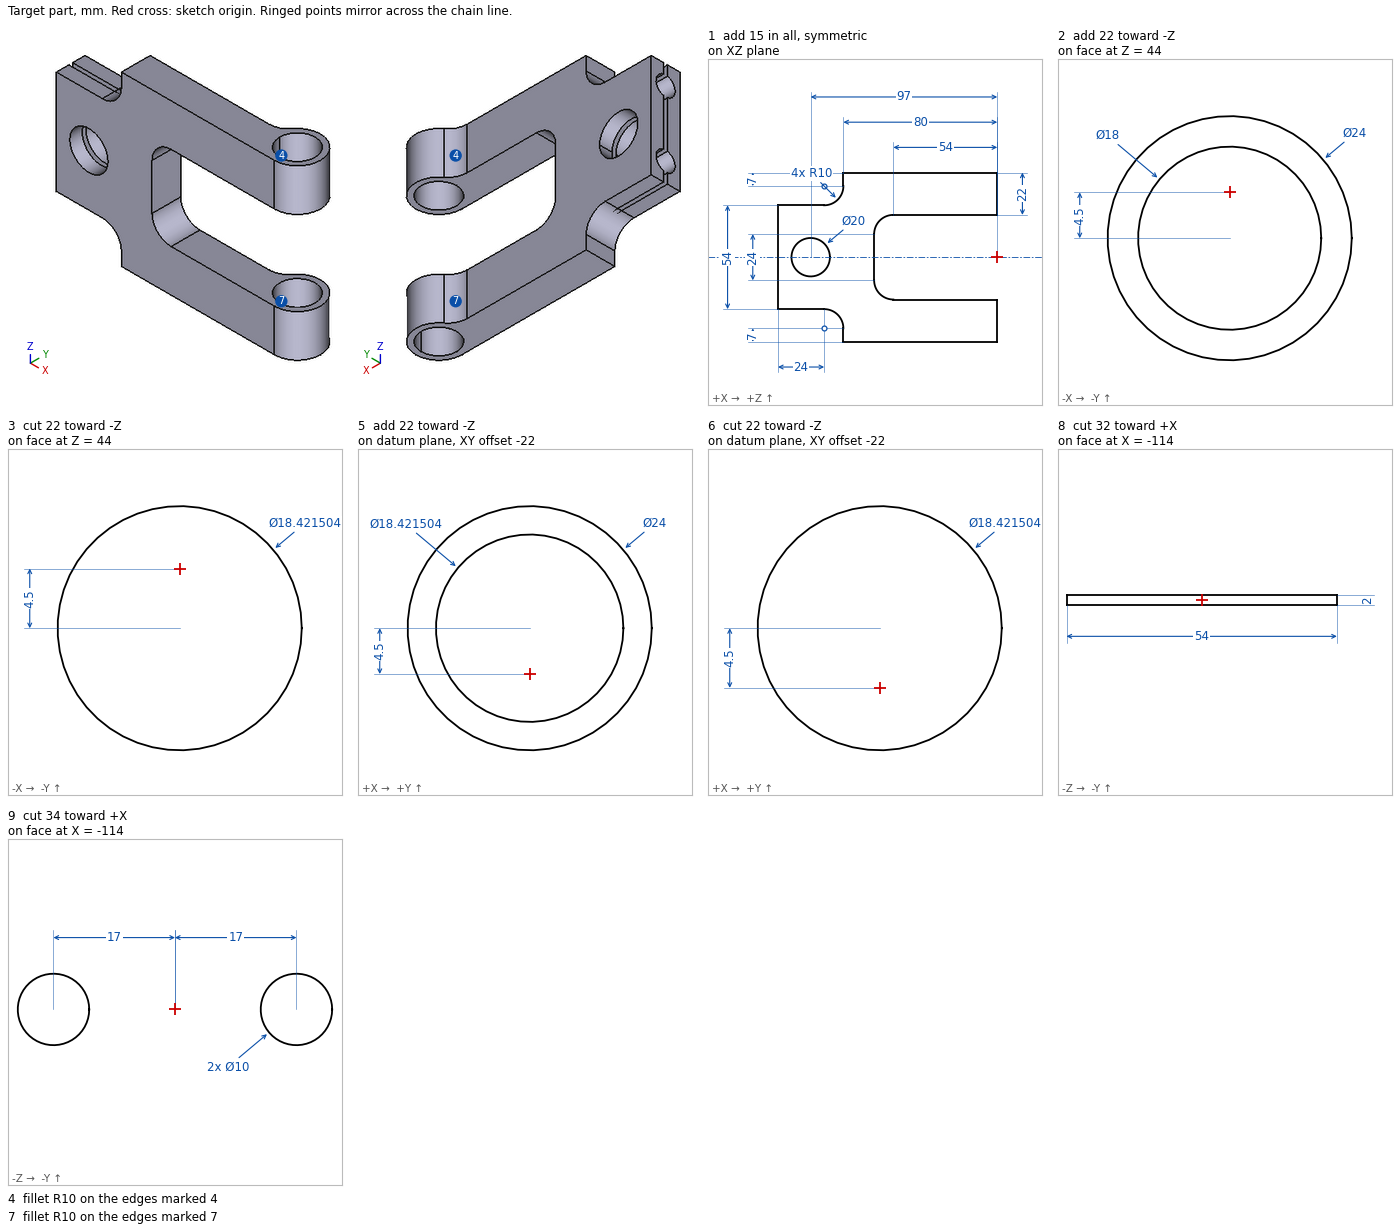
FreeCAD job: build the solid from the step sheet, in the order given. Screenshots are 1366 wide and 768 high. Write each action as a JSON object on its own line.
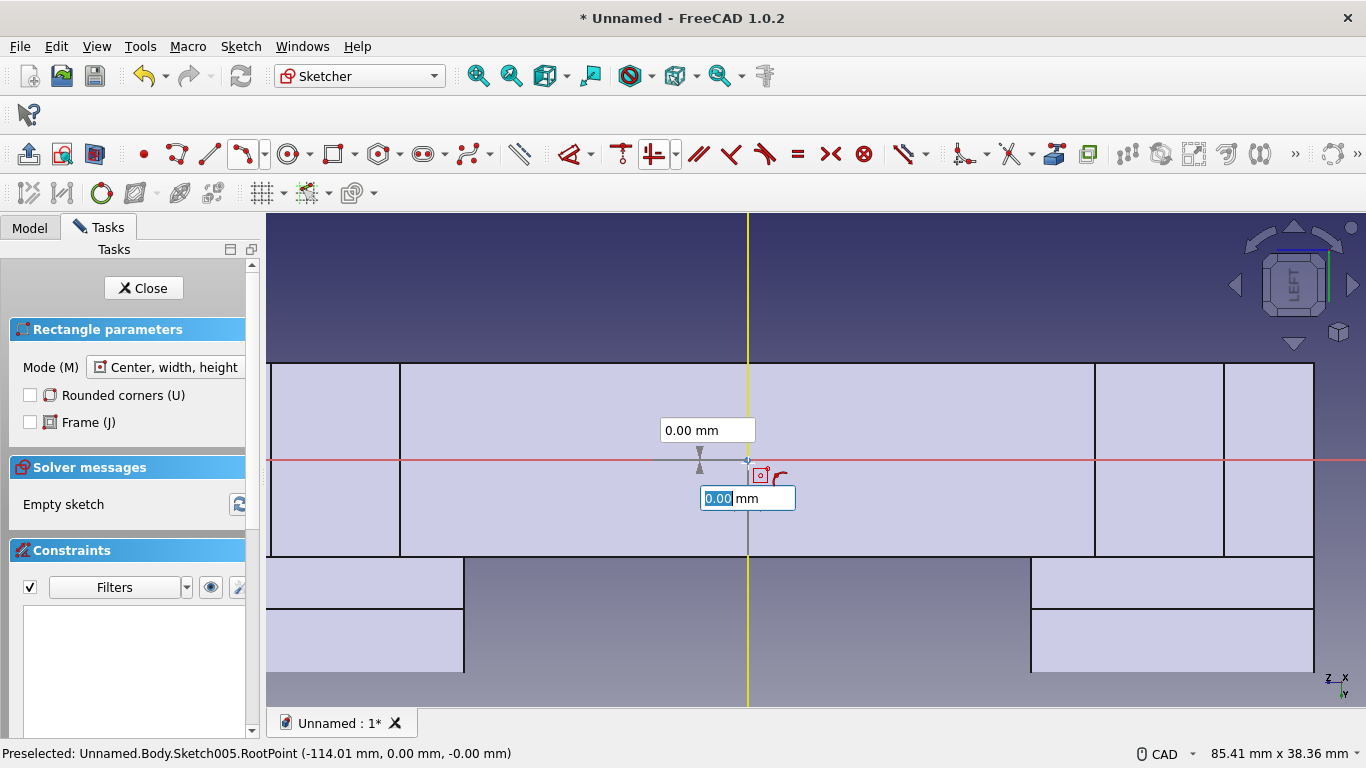
{"action": "scroll", "coordinate": [1095, 447], "scroll_direction": "up", "scroll_amount": 2}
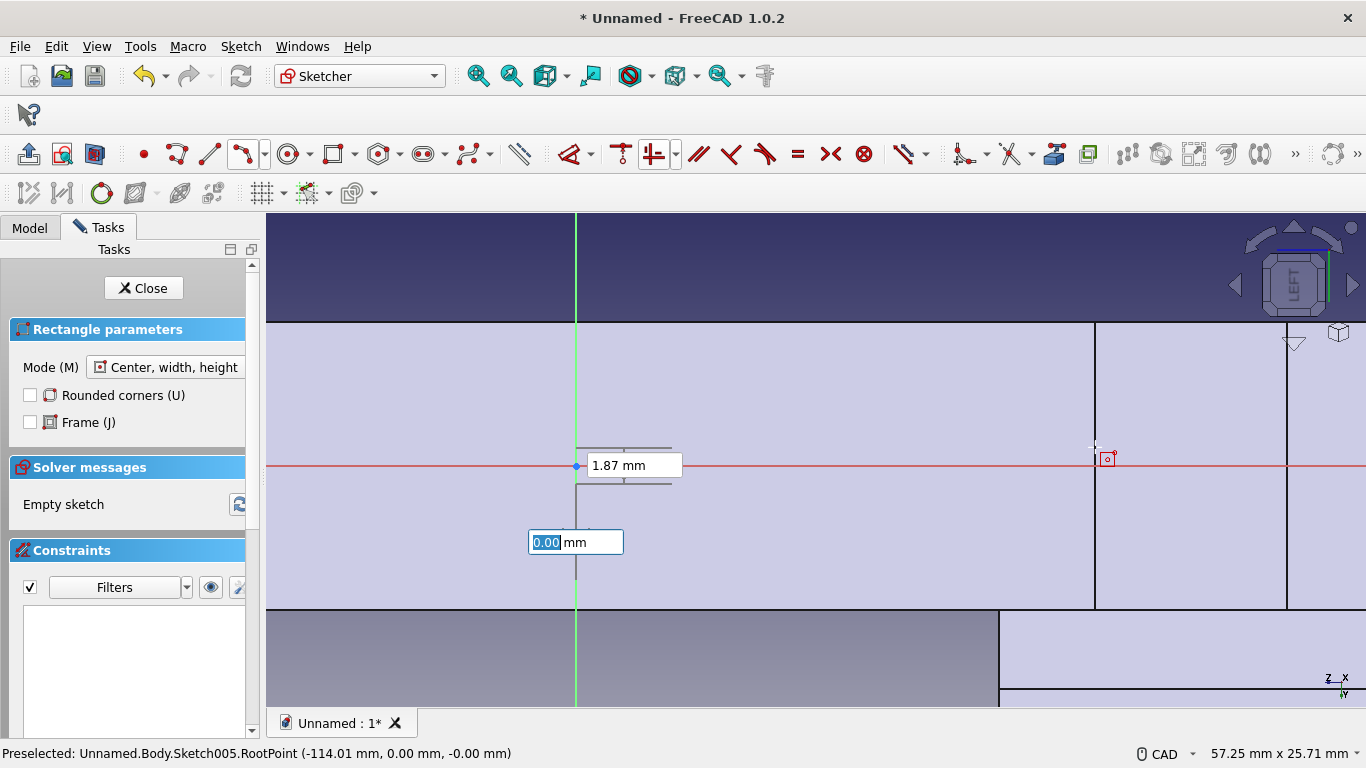
{"action": "left_click", "coordinate": [1095, 447]}
{"action": "key", "text": "Escape"}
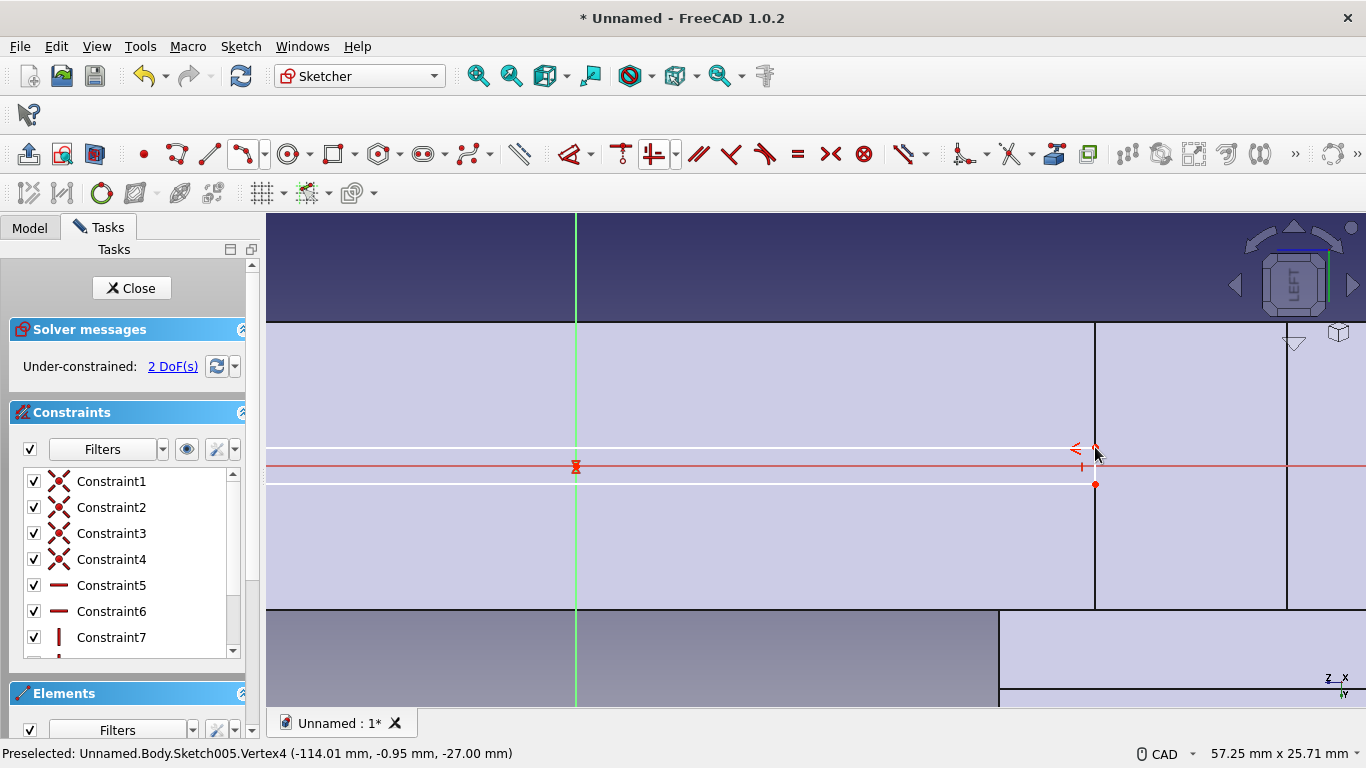
{"action": "left_click", "coordinate": [568, 154]}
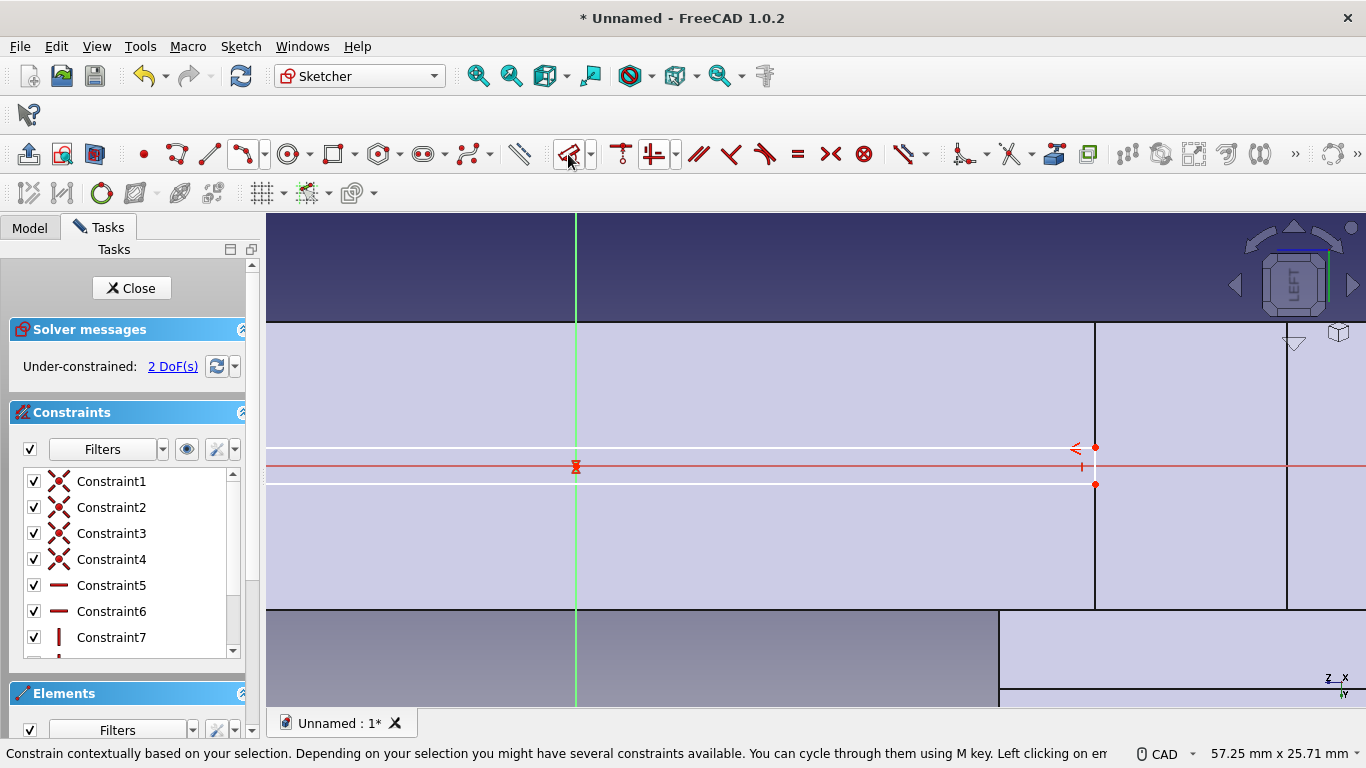
{"action": "left_click", "coordinate": [1095, 470]}
{"action": "left_click", "coordinate": [1129, 458]}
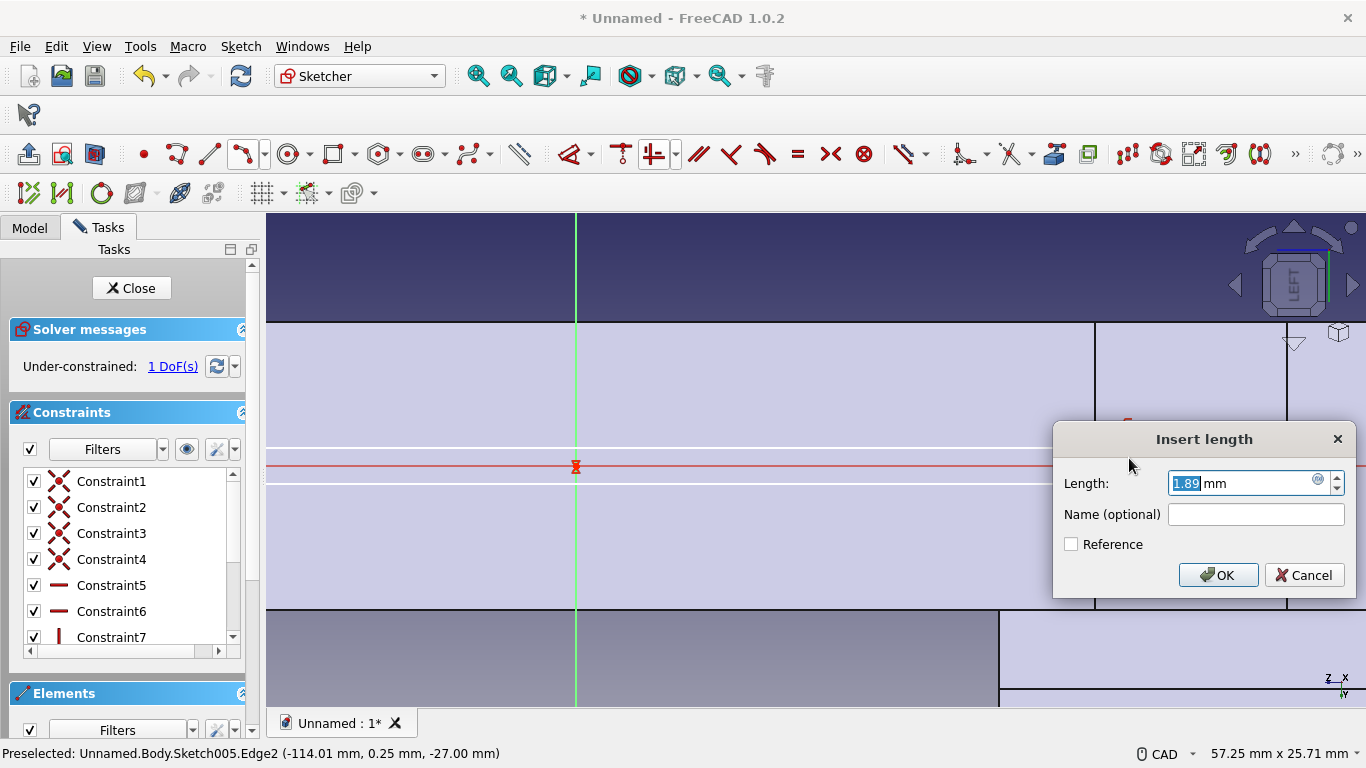
{"action": "type", "text": "2"}
{"action": "key", "text": "Return"}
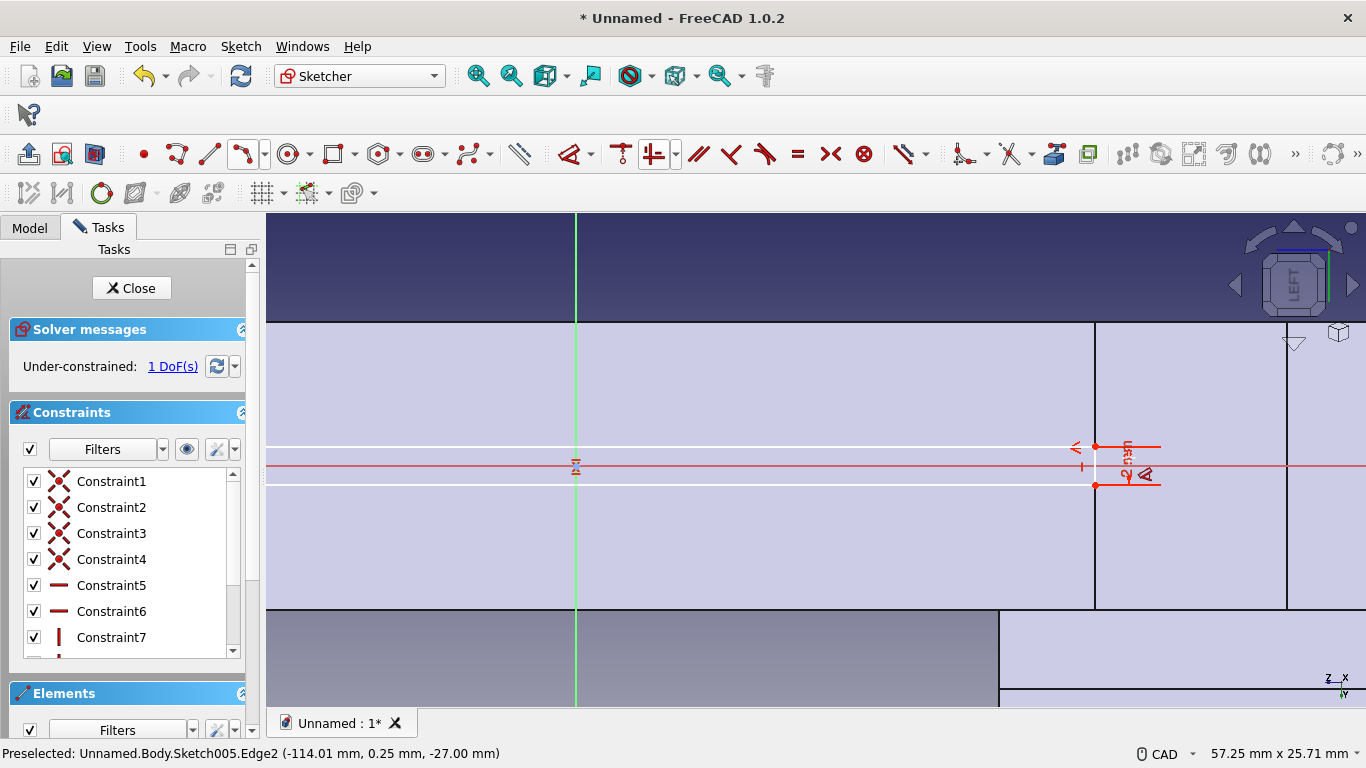
{"action": "left_click", "coordinate": [369, 485]}
{"action": "left_click", "coordinate": [695, 519]}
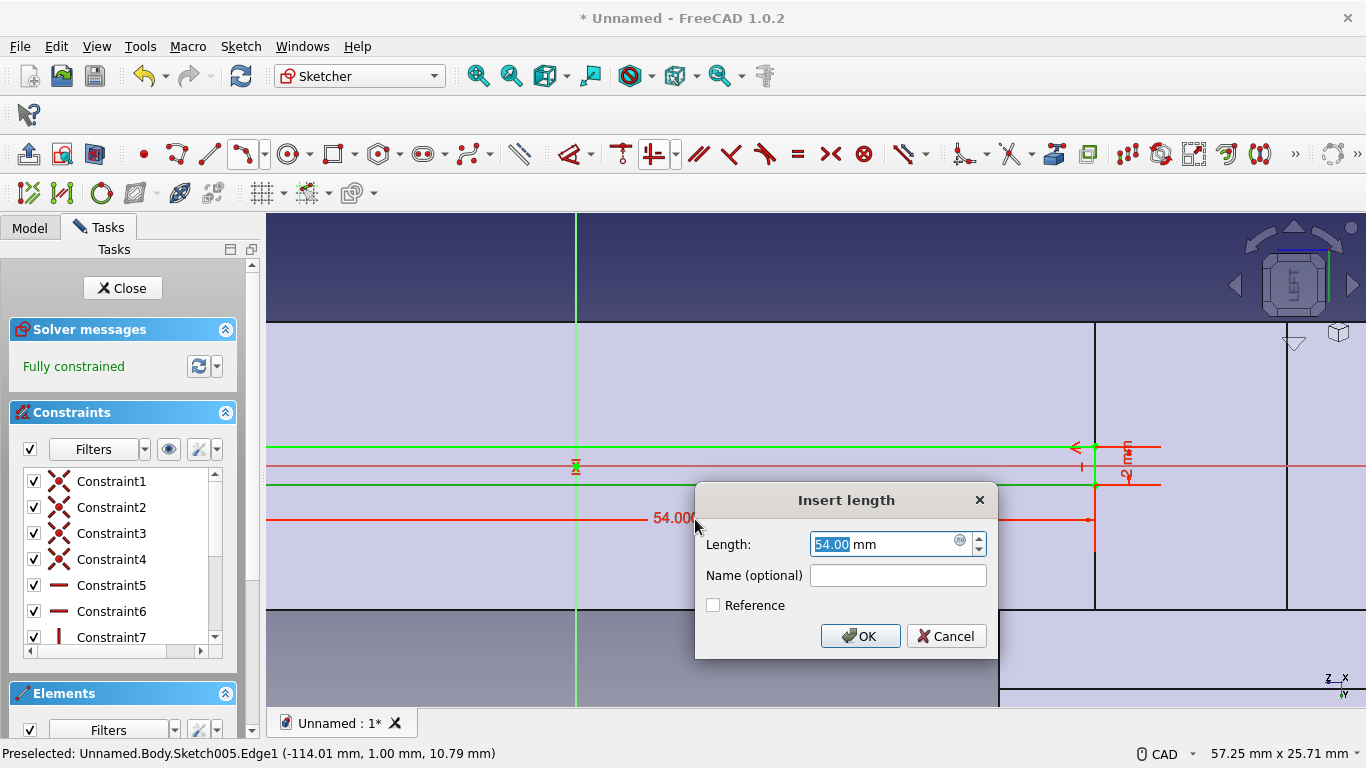
{"action": "type", "text": "54"}
{"action": "key", "text": "Return"}
{"action": "key", "text": "Escape"}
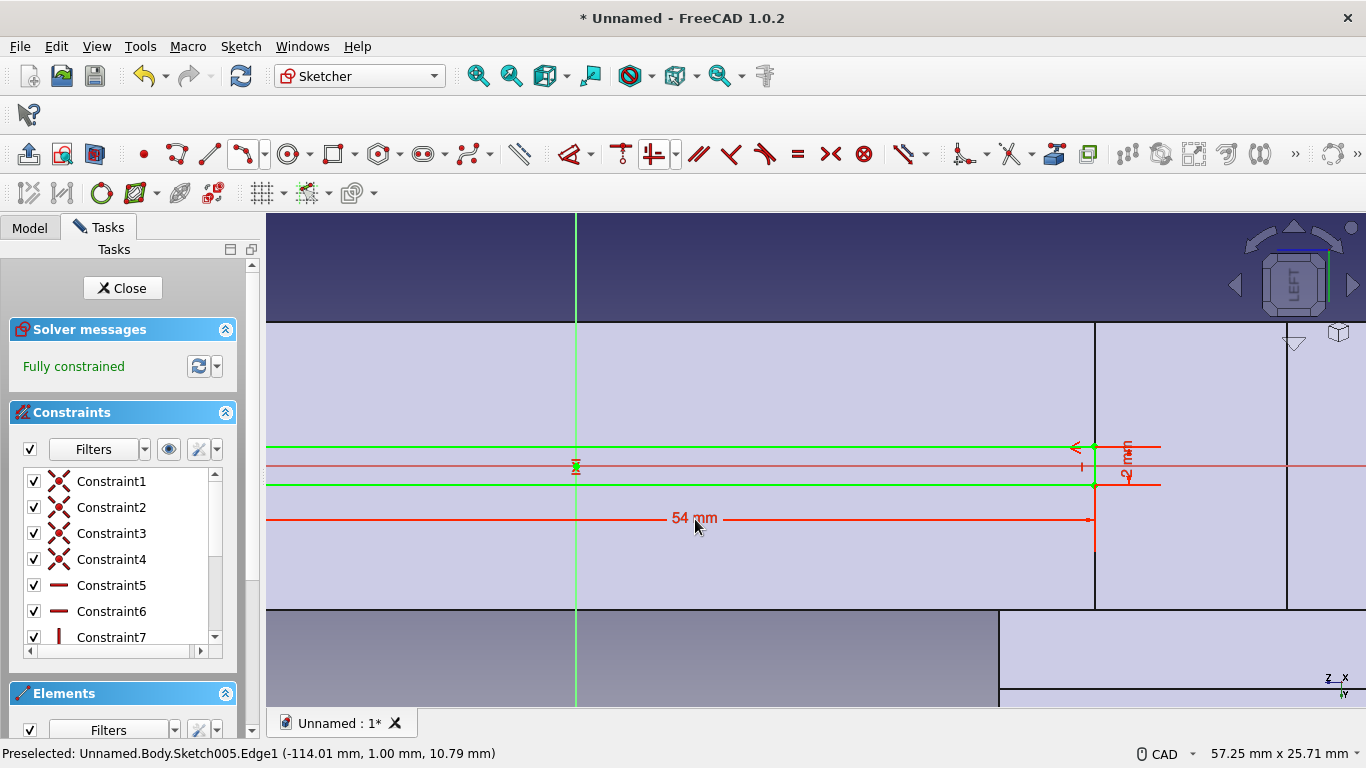
{"action": "left_click", "coordinate": [123, 288]}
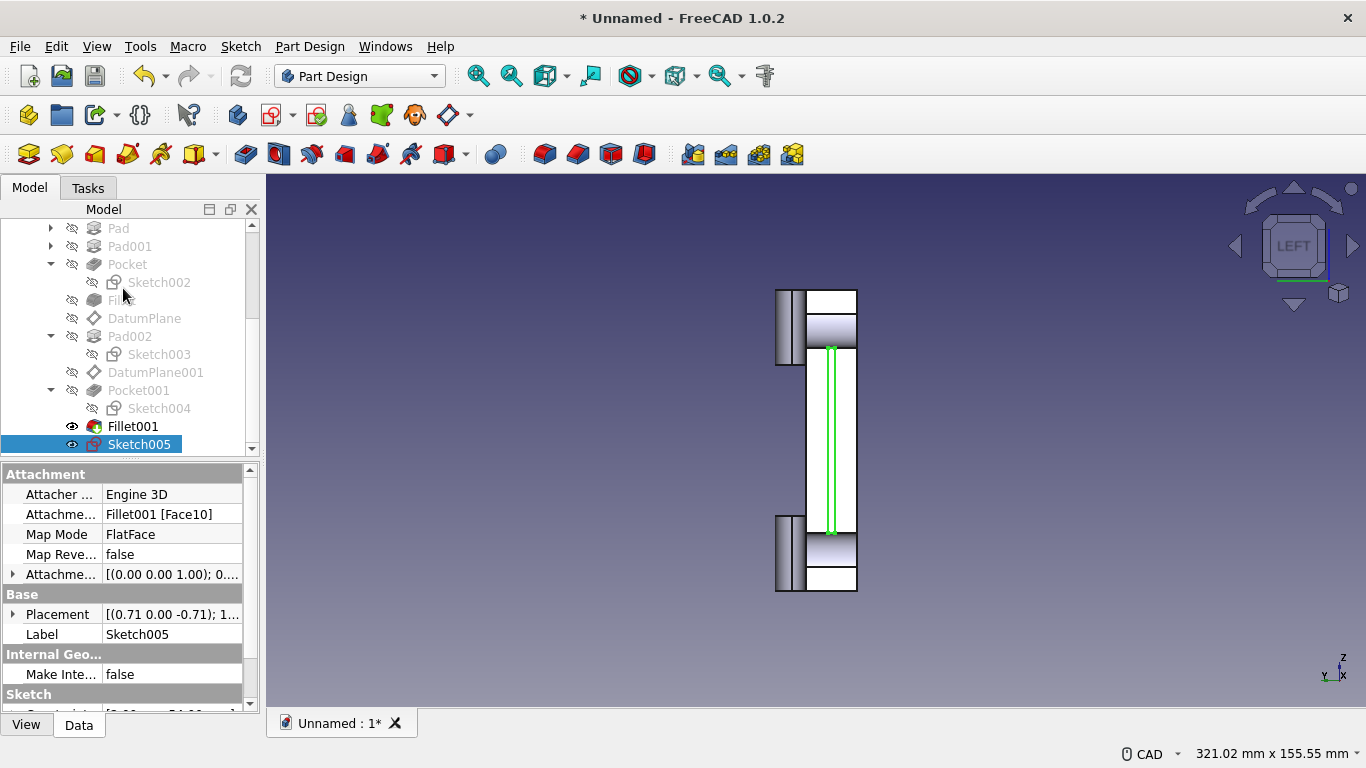
{"action": "left_click", "coordinate": [246, 154]}